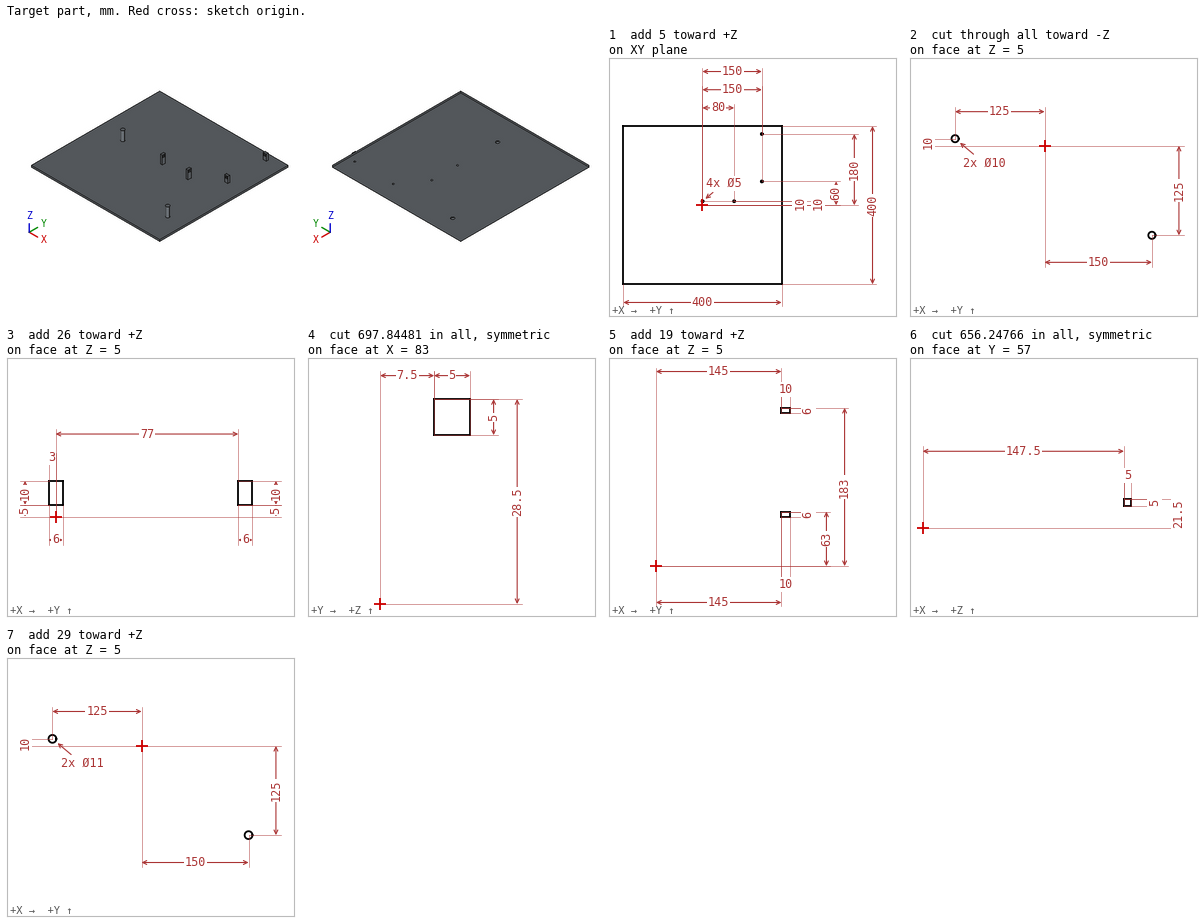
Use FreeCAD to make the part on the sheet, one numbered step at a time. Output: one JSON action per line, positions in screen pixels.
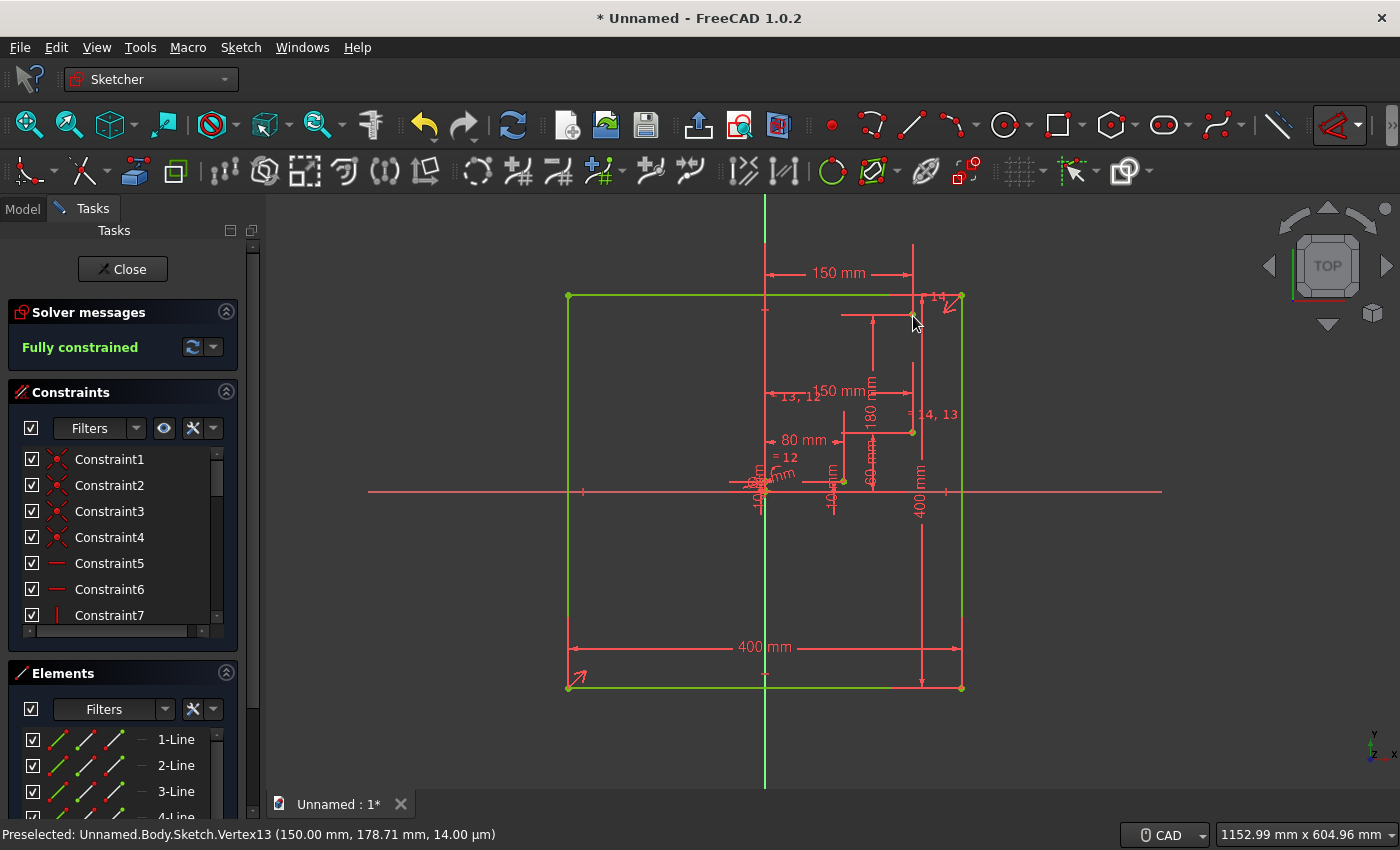
{"action": "left_click", "coordinate": [123, 269]}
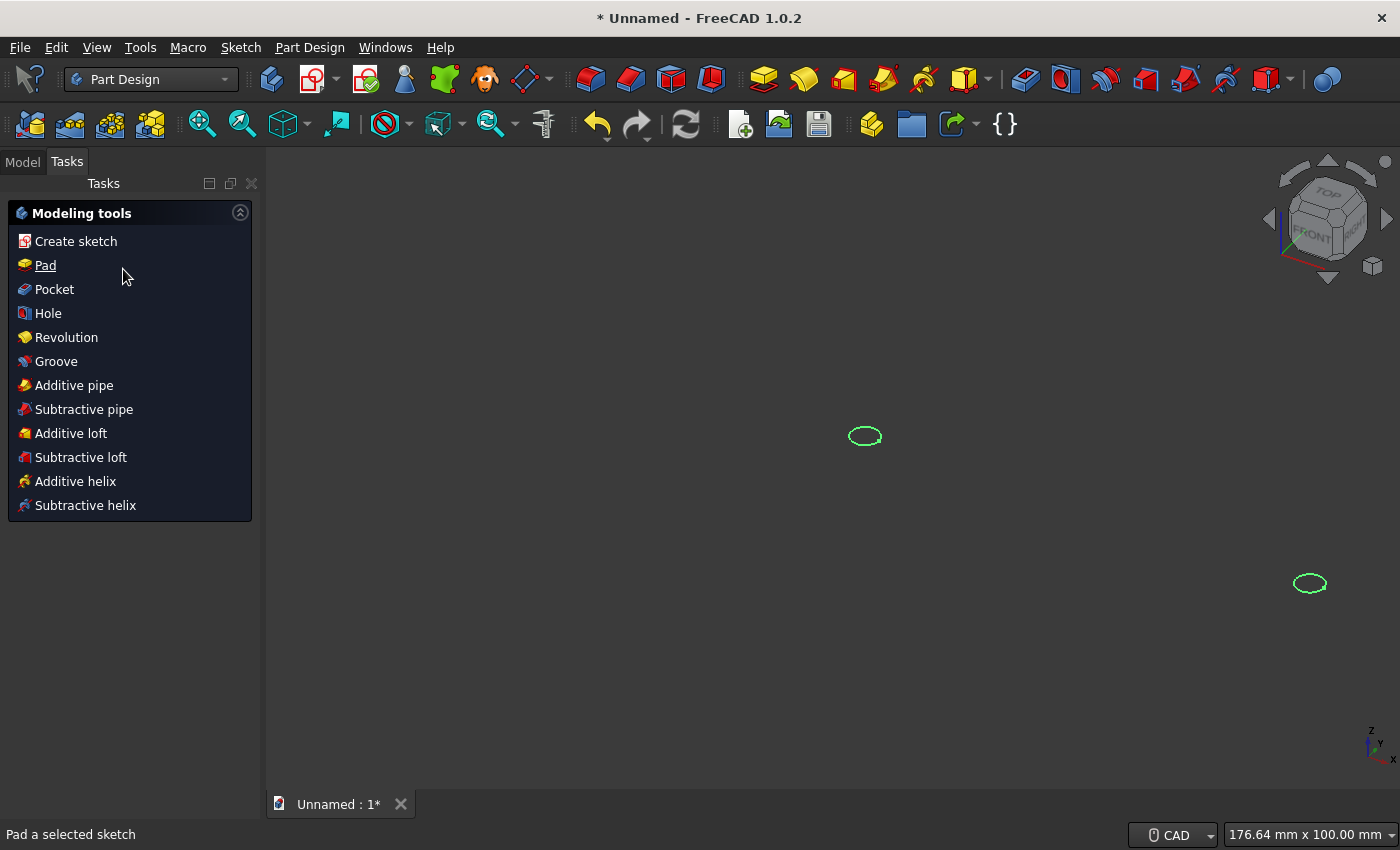
{"action": "left_click", "coordinate": [764, 80]}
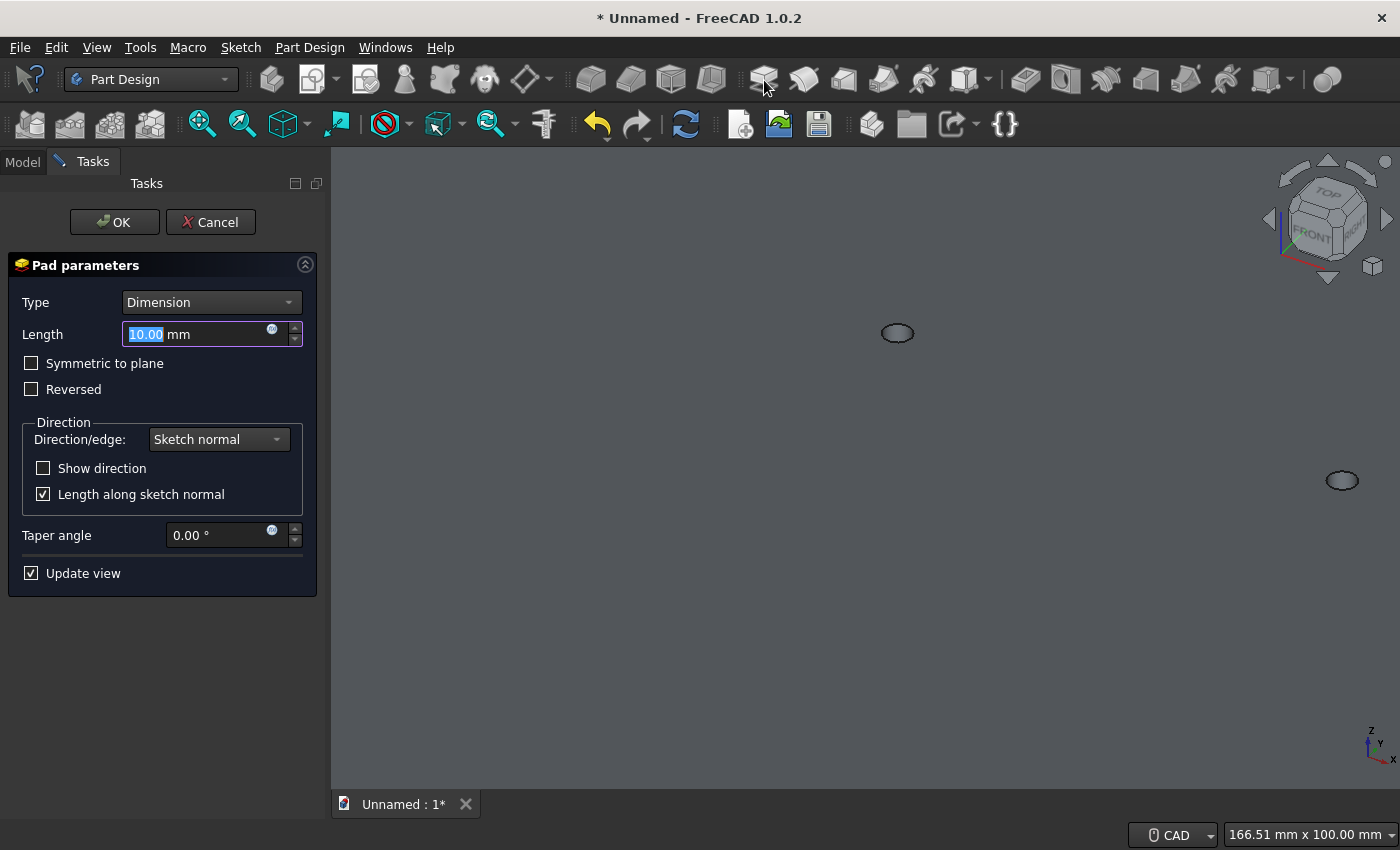
{"action": "type", "text": "5"}
{"action": "key", "text": "Tab"}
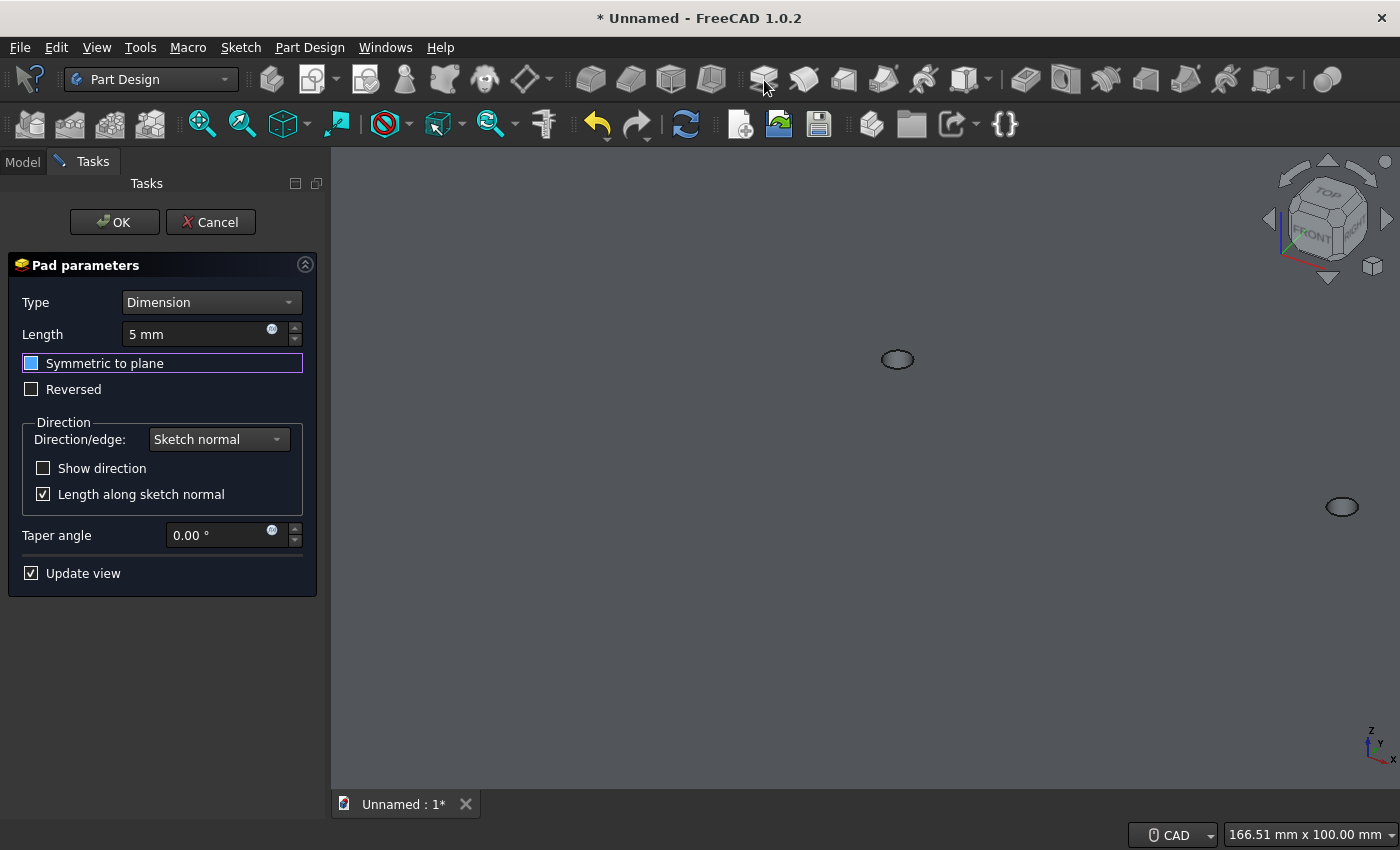
{"action": "left_click", "coordinate": [115, 222]}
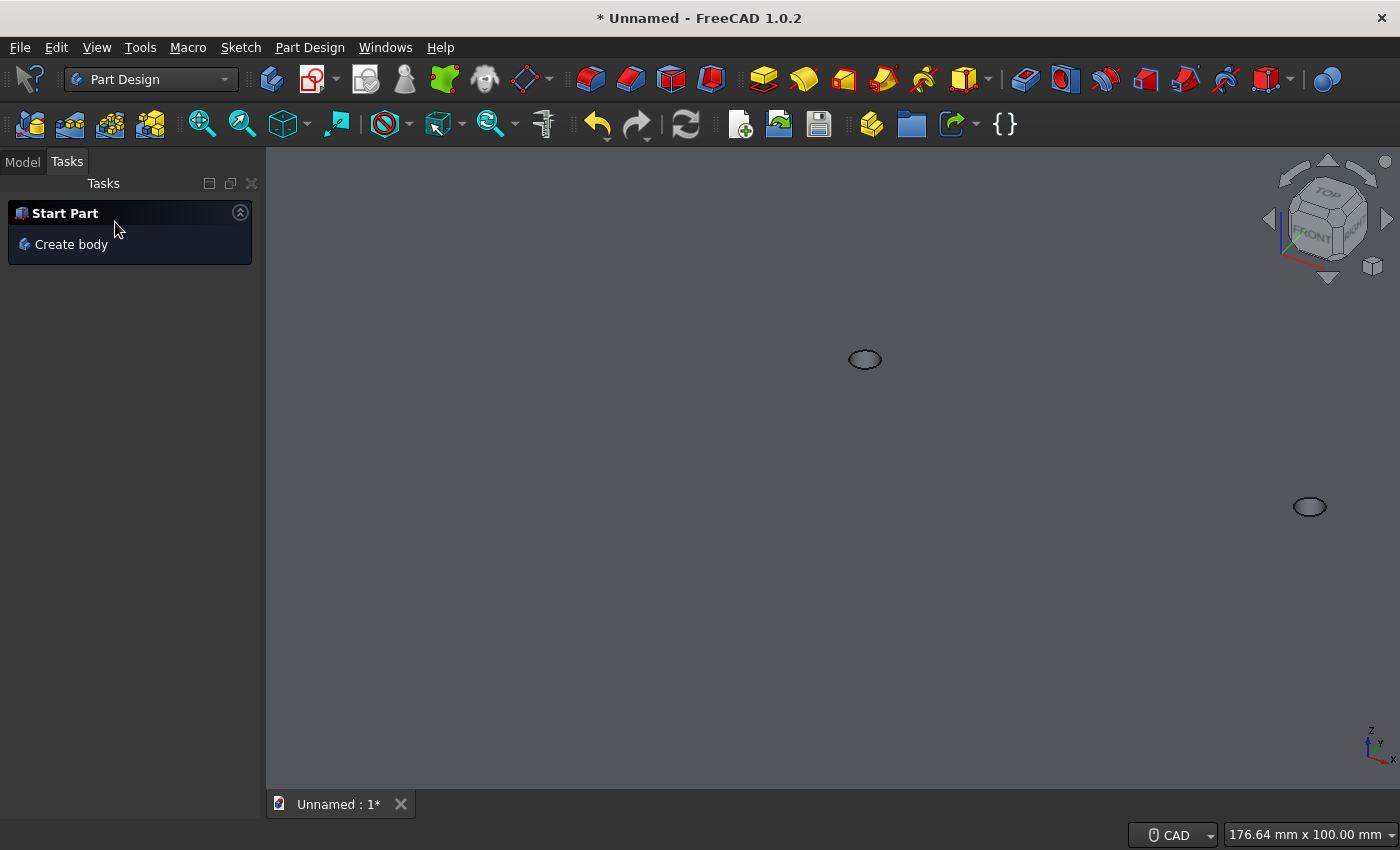
{"action": "key", "text": "v f"}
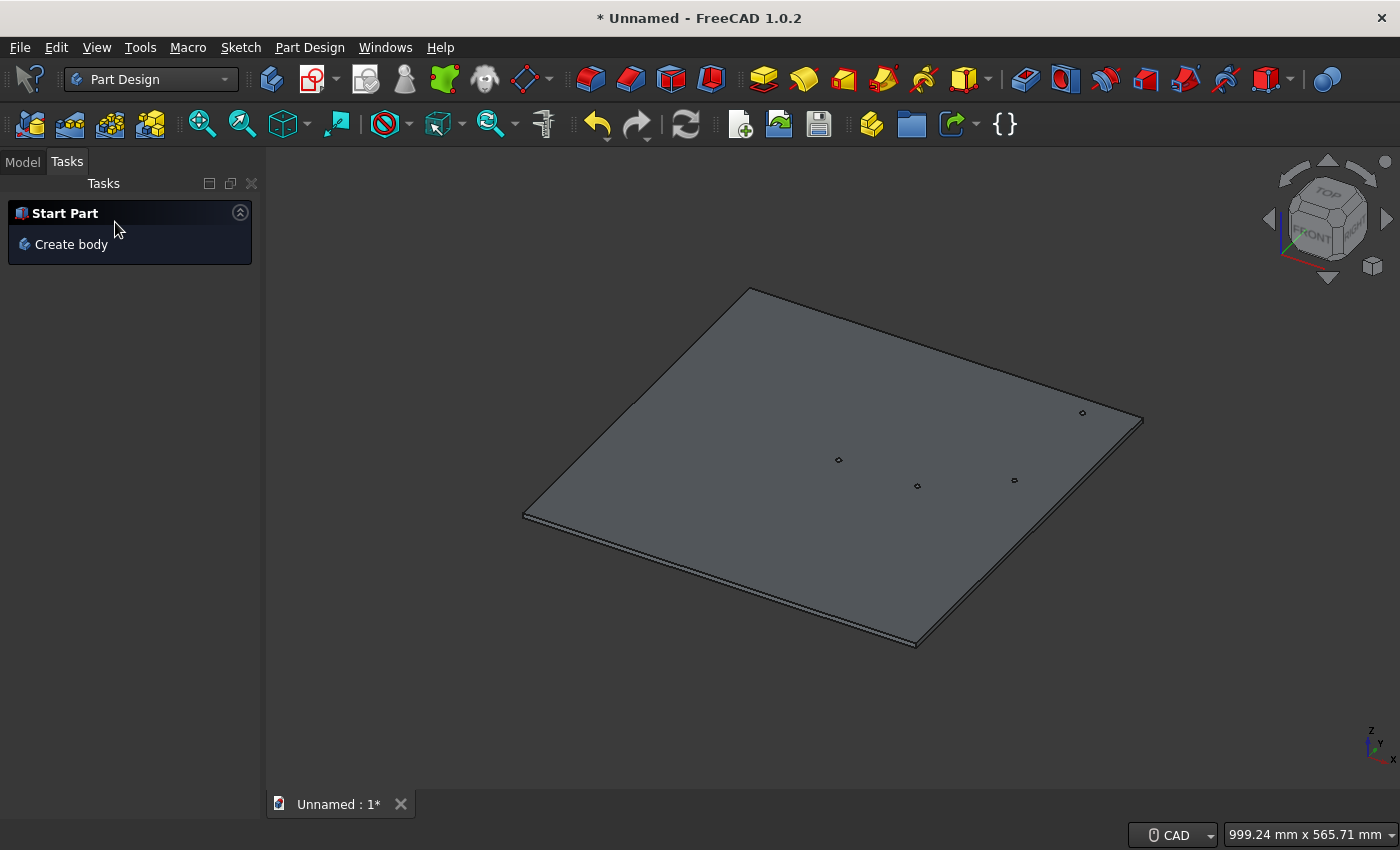
{"action": "left_click", "coordinate": [954, 419]}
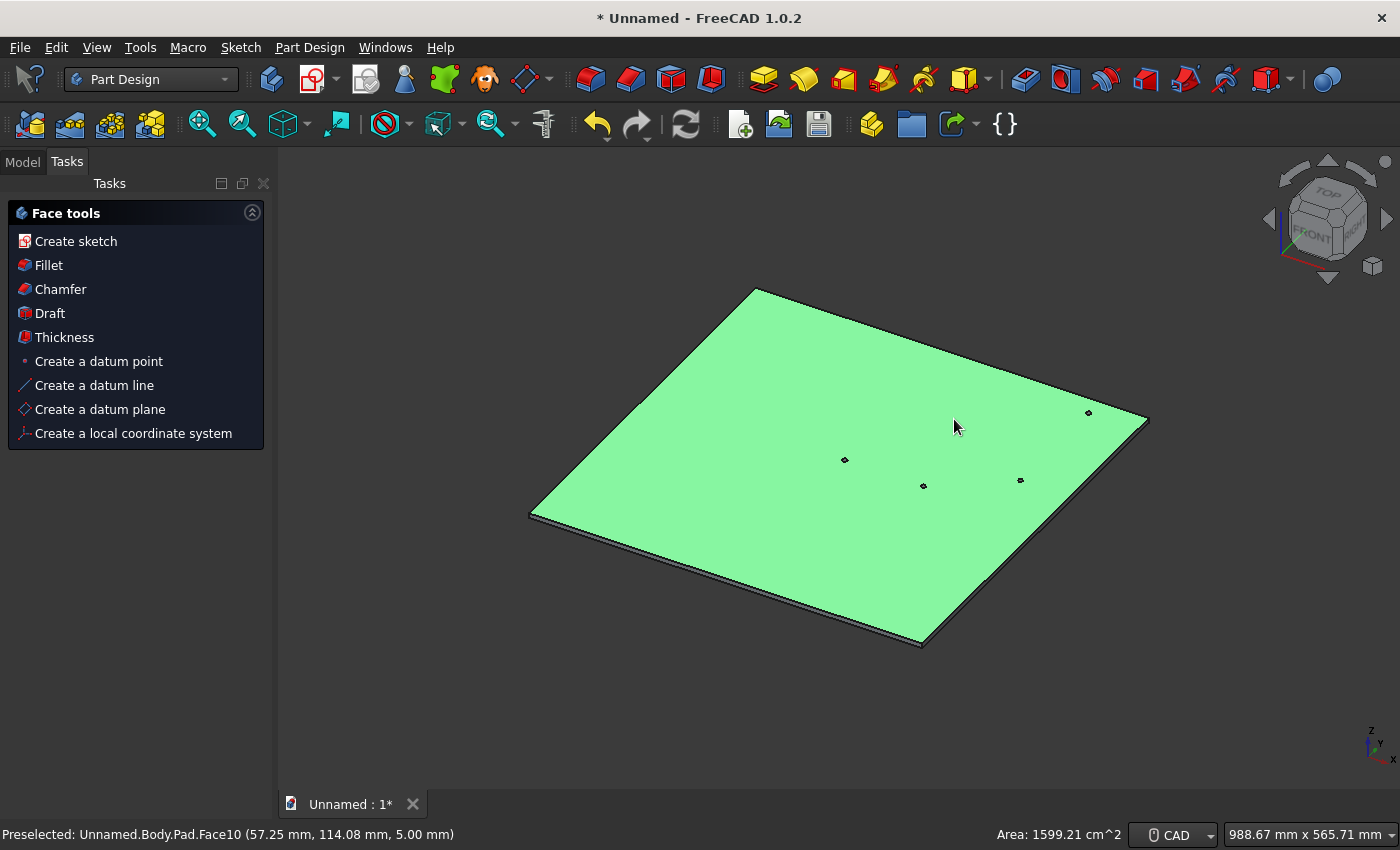
{"action": "left_click", "coordinate": [312, 80]}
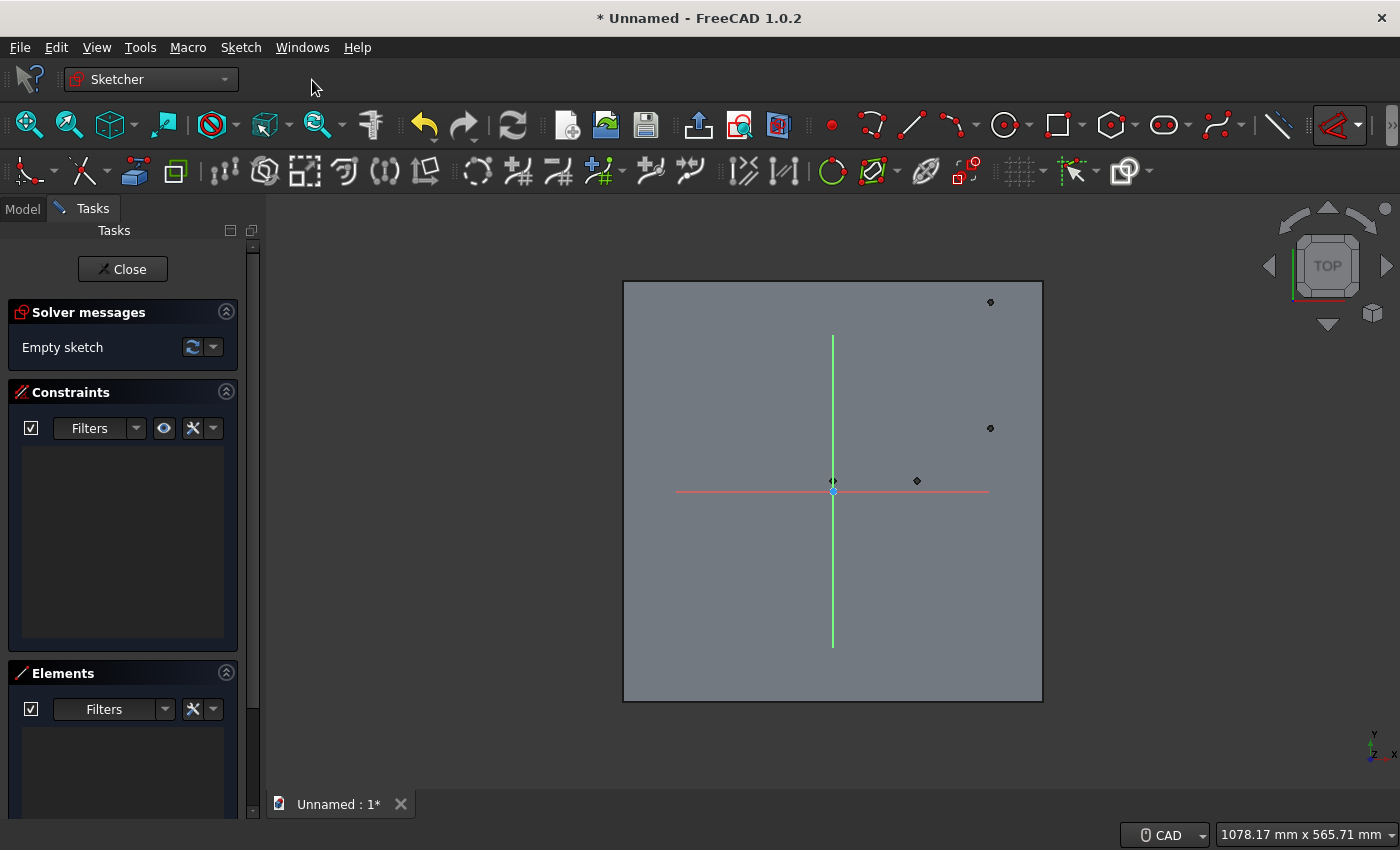
{"action": "scroll", "coordinate": [913, 601], "scroll_direction": "up", "scroll_amount": 4}